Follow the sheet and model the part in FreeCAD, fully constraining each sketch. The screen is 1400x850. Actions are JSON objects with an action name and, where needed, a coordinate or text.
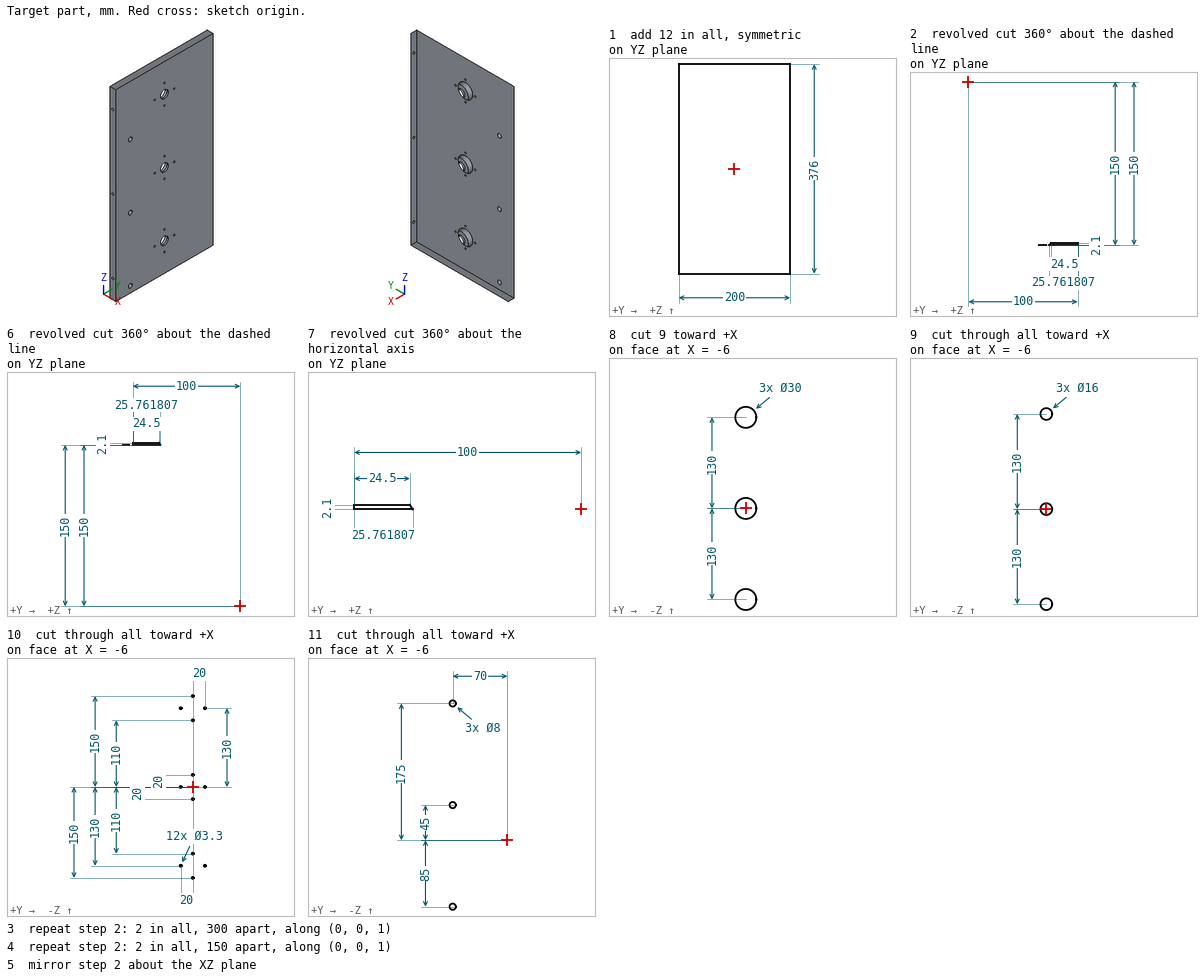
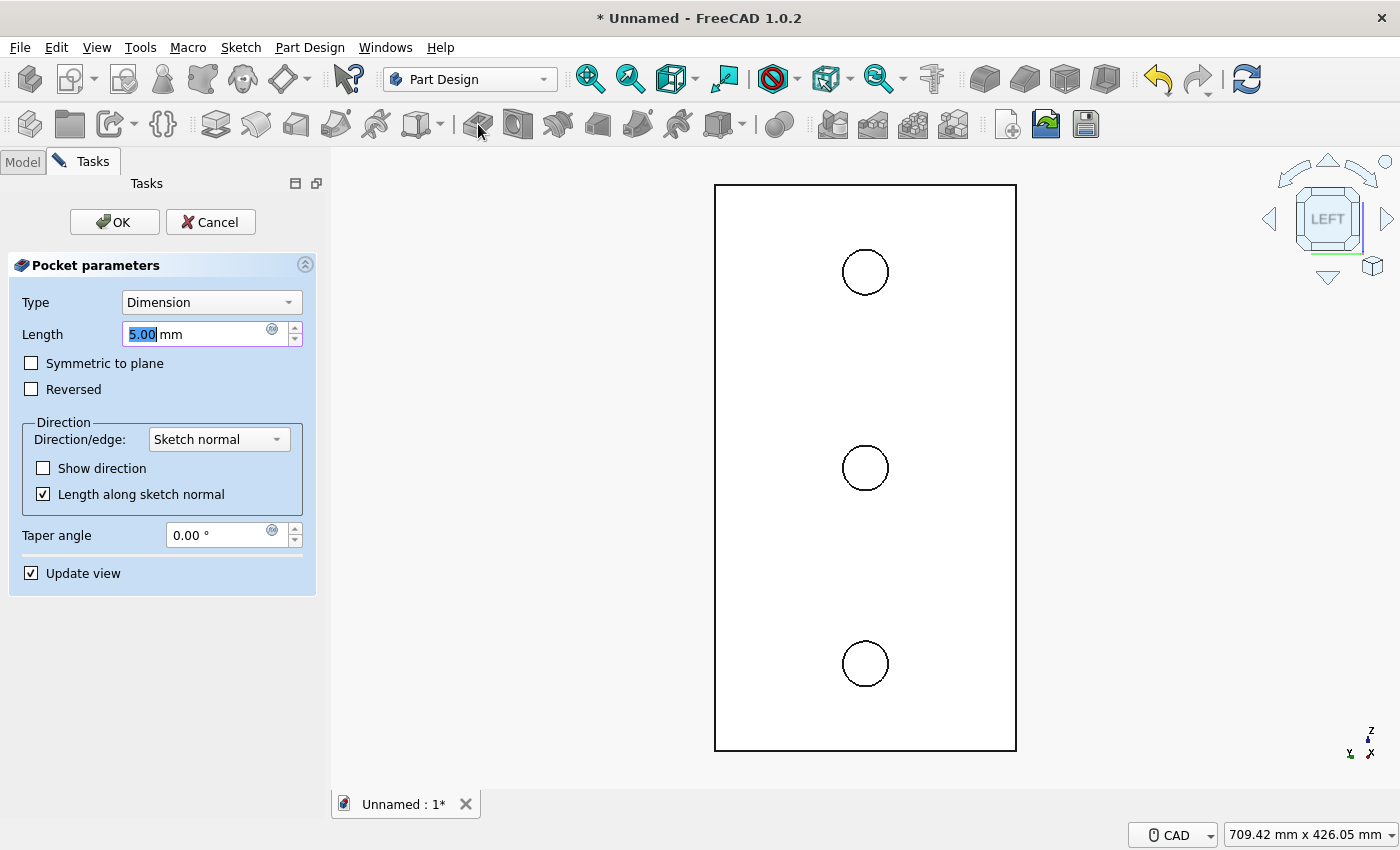
{"action": "left_click", "coordinate": [212, 302]}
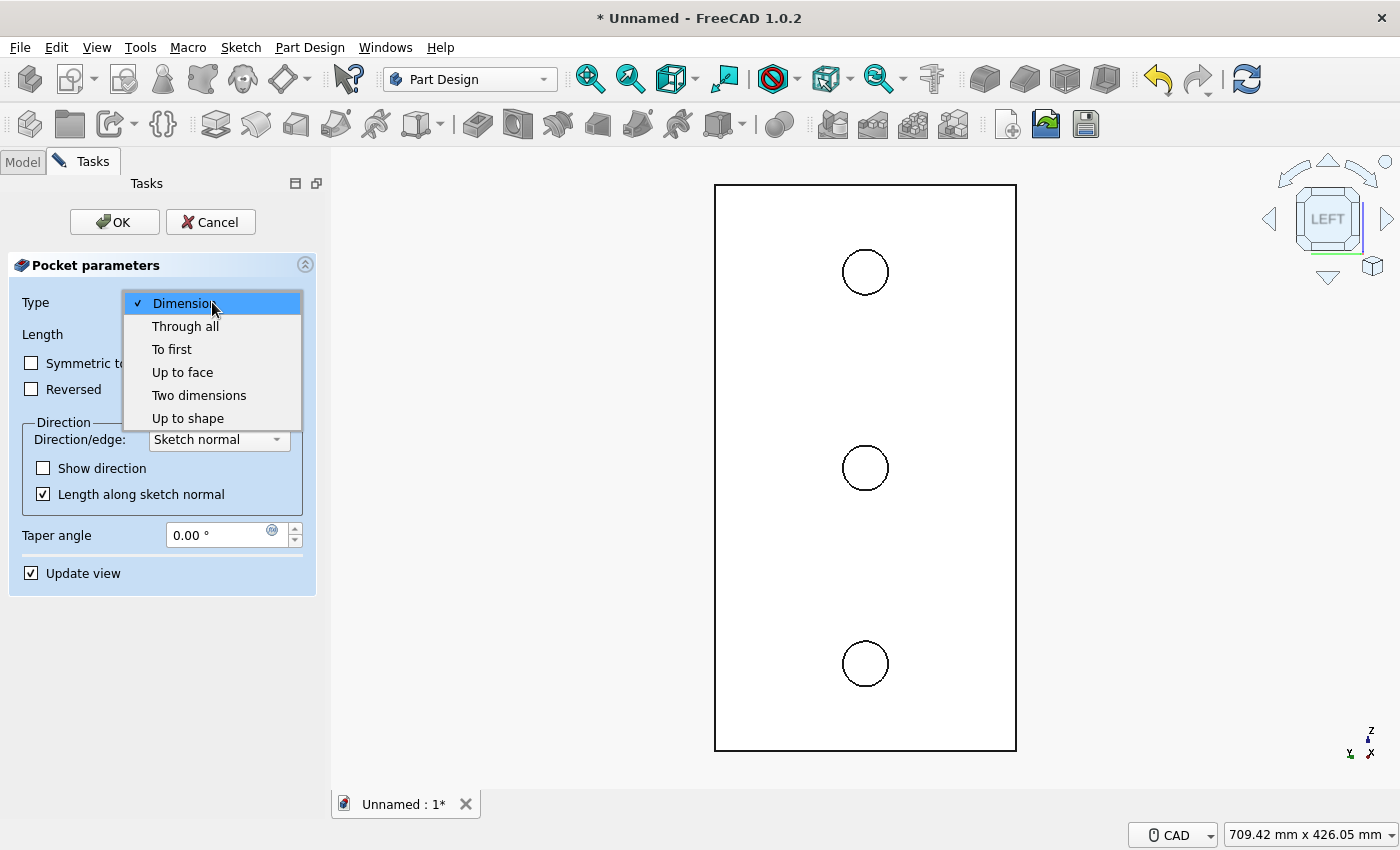
{"action": "left_click", "coordinate": [212, 326]}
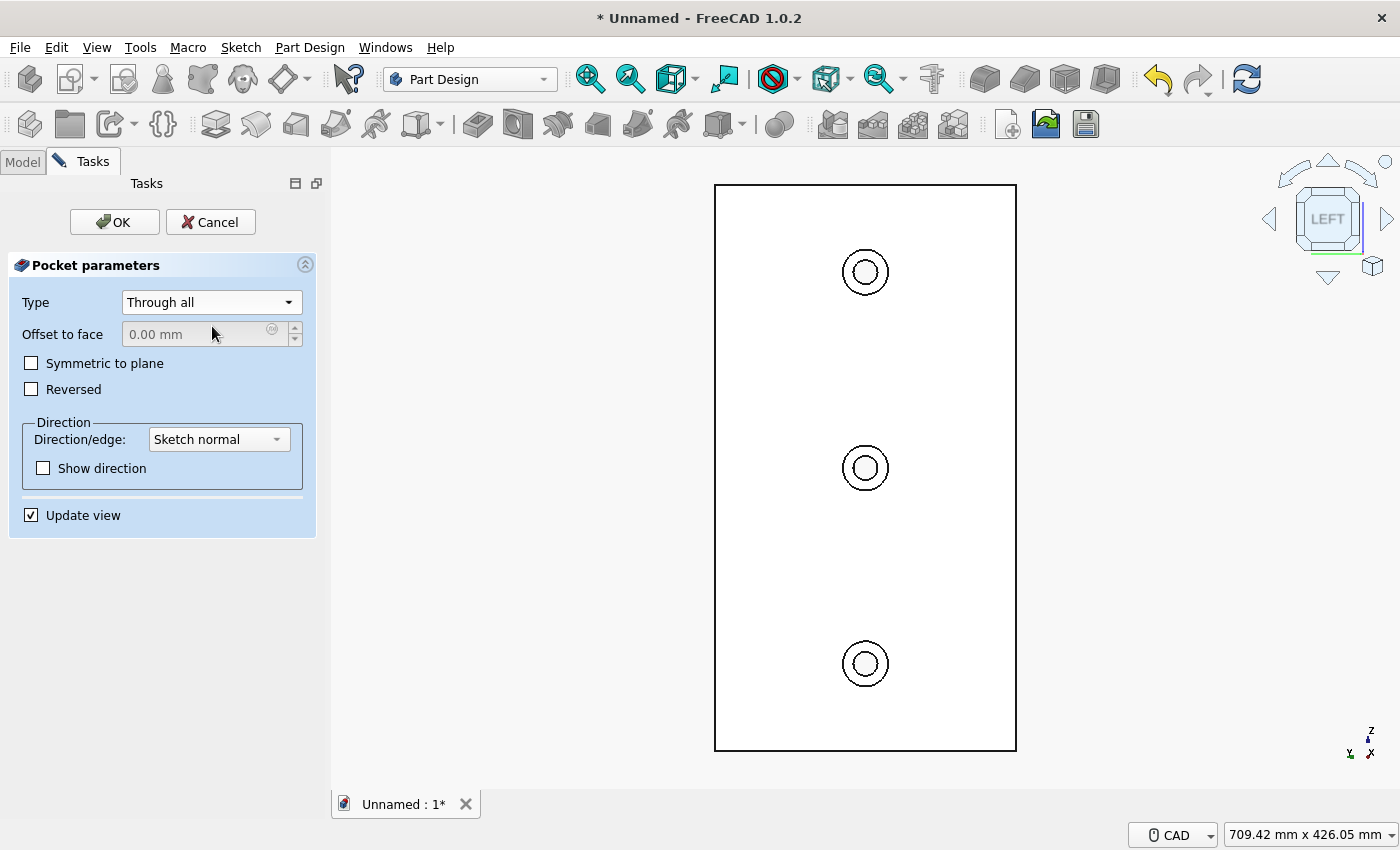
{"action": "left_click", "coordinate": [115, 222]}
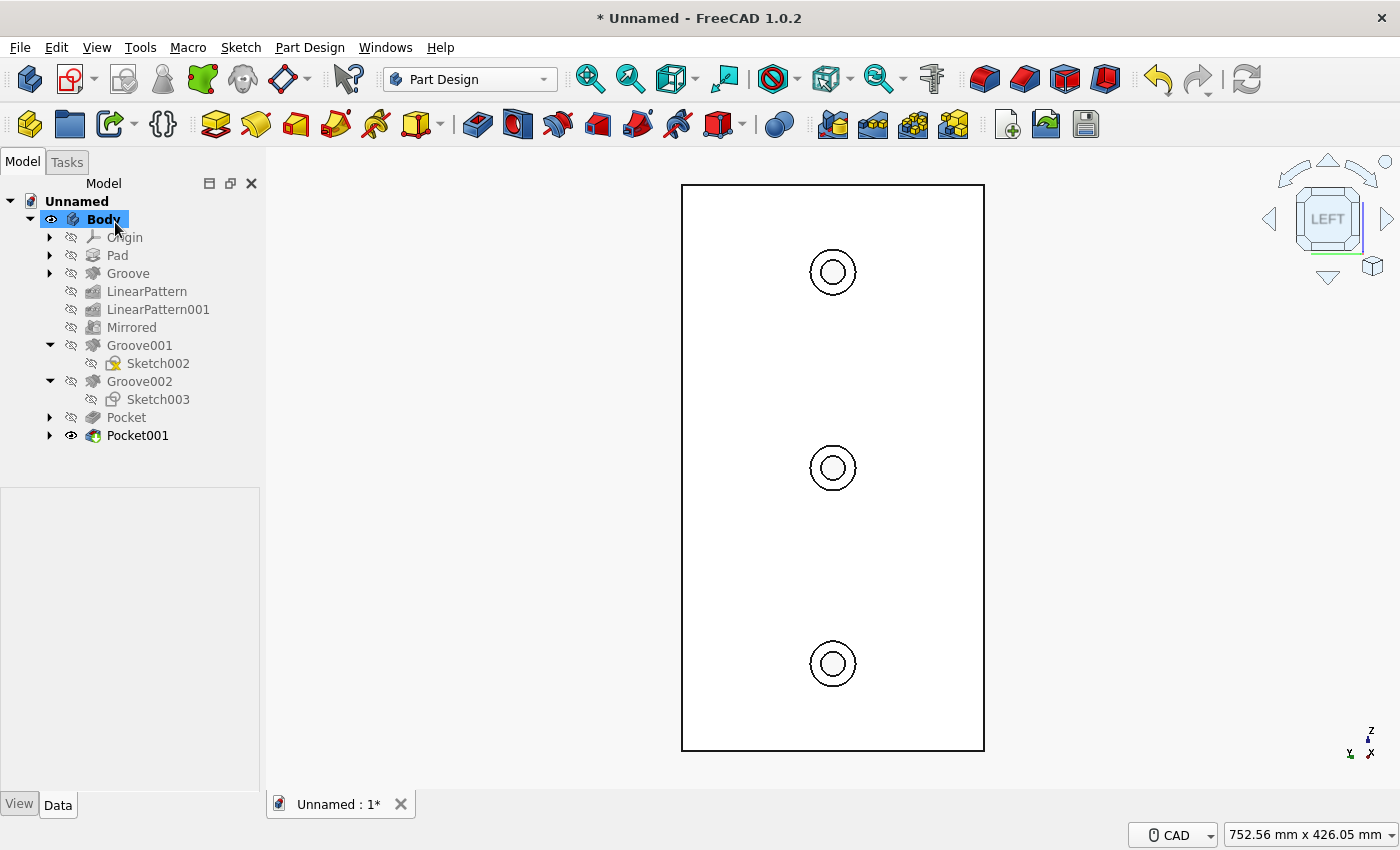
{"action": "left_click", "coordinate": [790, 548]}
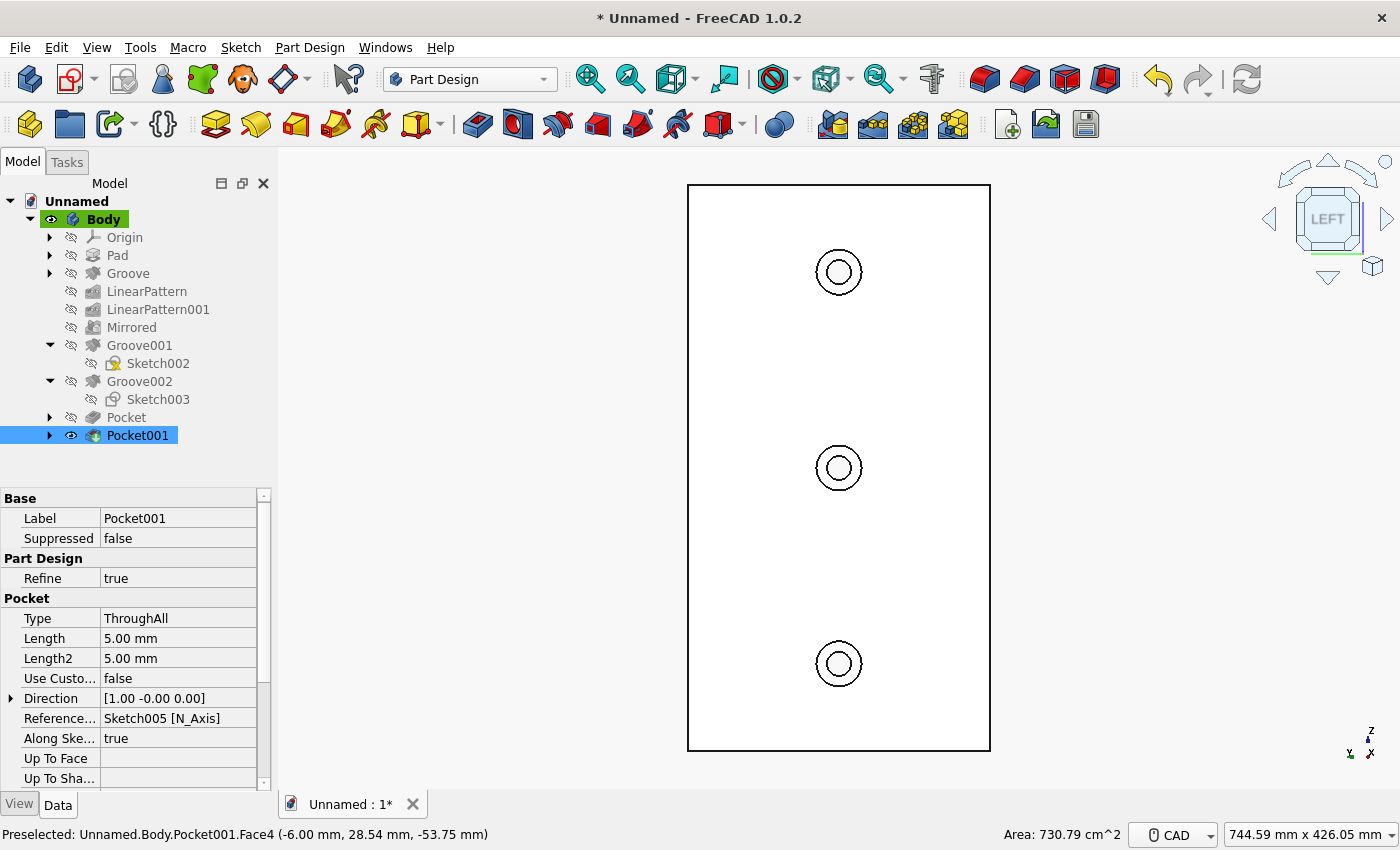
{"action": "left_click", "coordinate": [70, 80]}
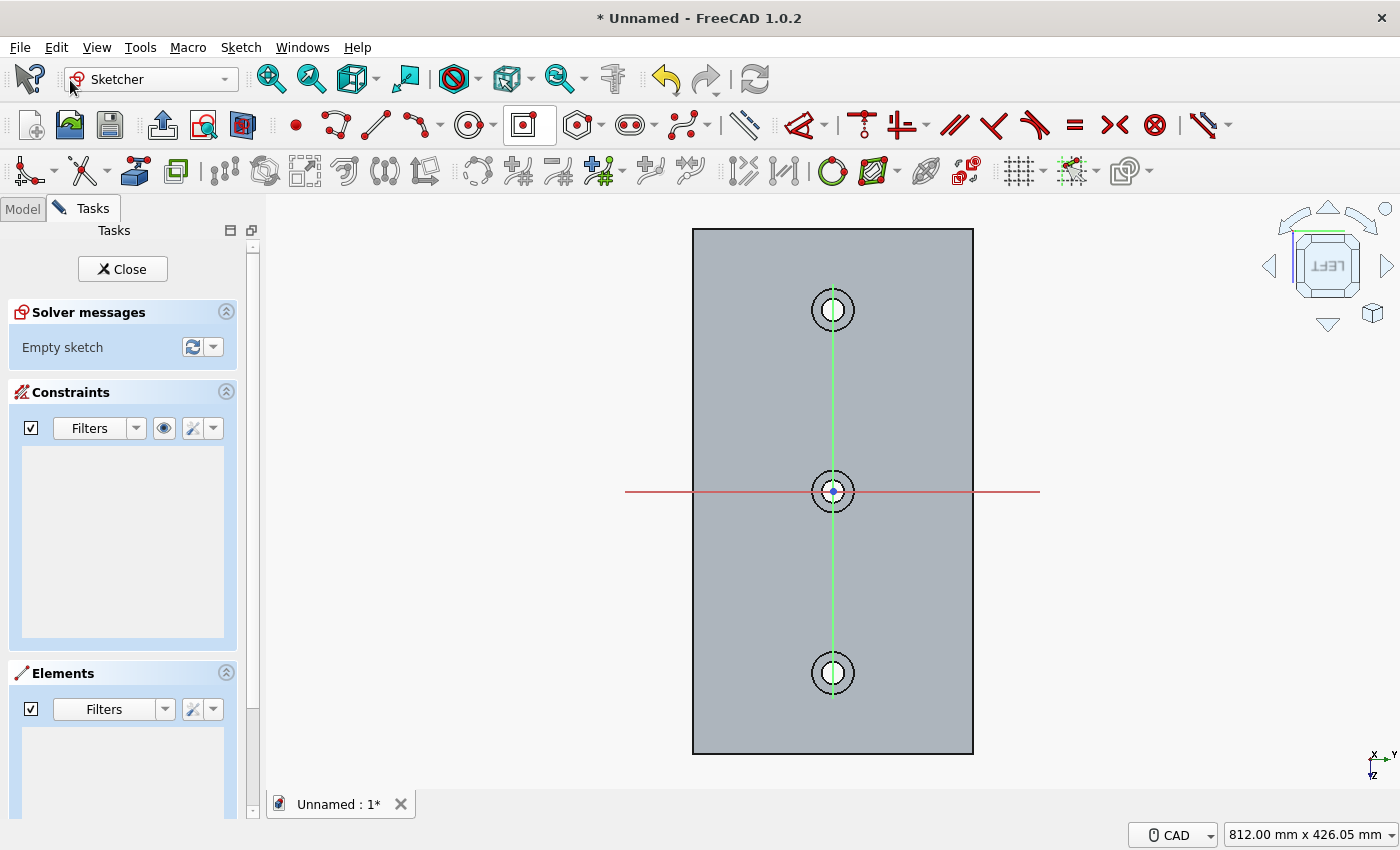
{"action": "left_click", "coordinate": [470, 126]}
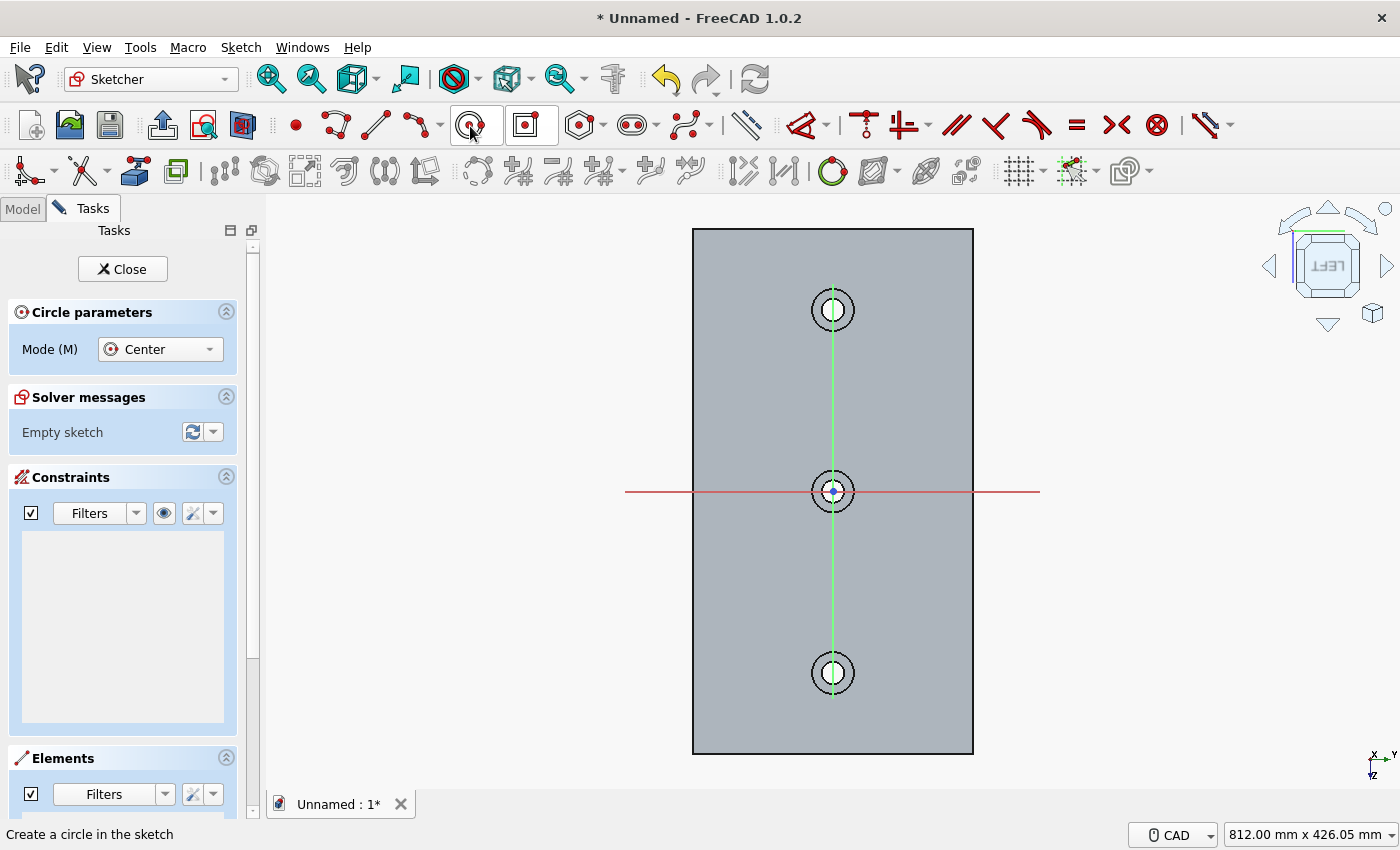
{"action": "scroll", "coordinate": [805, 673], "scroll_direction": "up", "scroll_amount": 12}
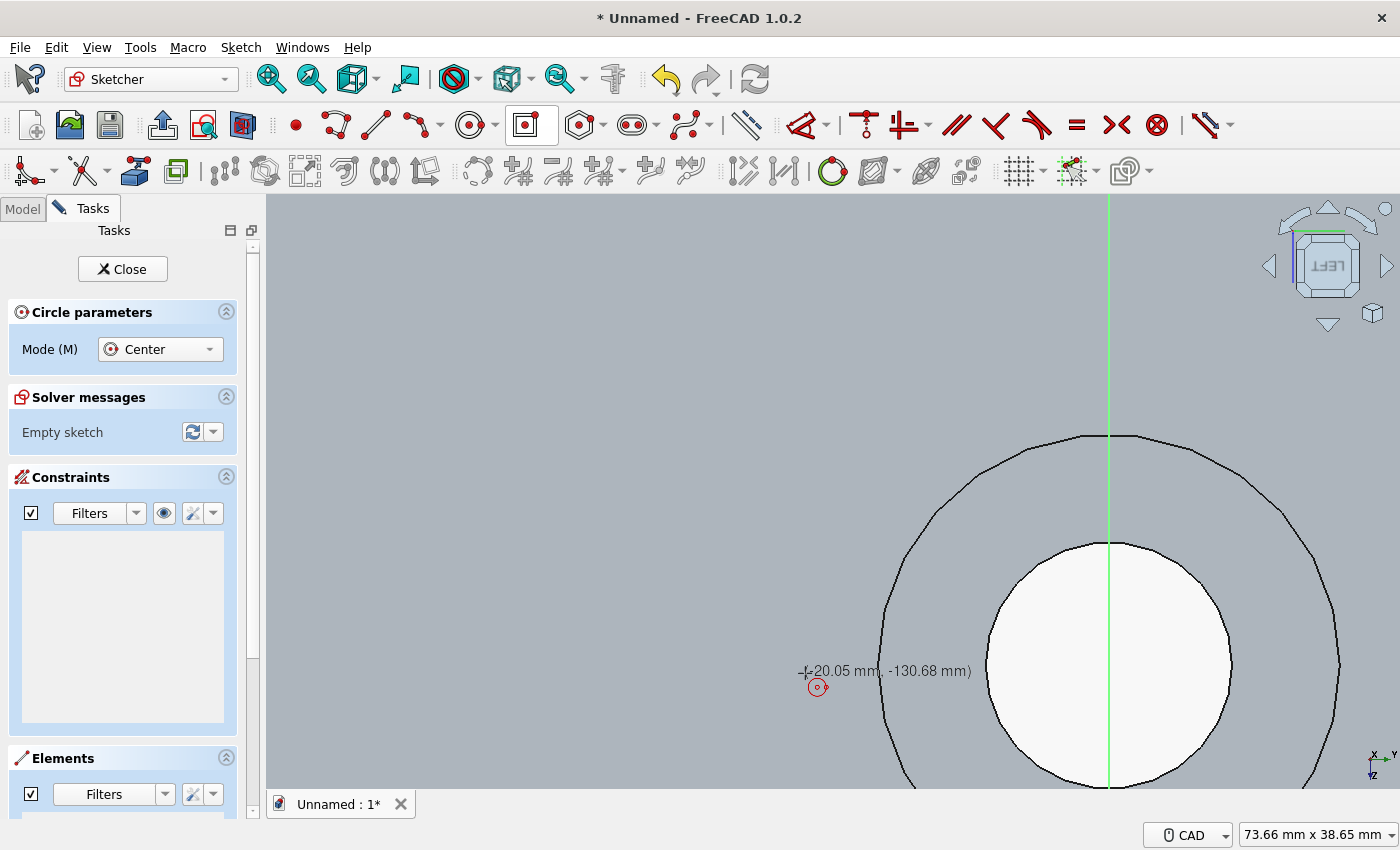
{"action": "scroll", "coordinate": [737, 638], "scroll_direction": "down", "scroll_amount": 13}